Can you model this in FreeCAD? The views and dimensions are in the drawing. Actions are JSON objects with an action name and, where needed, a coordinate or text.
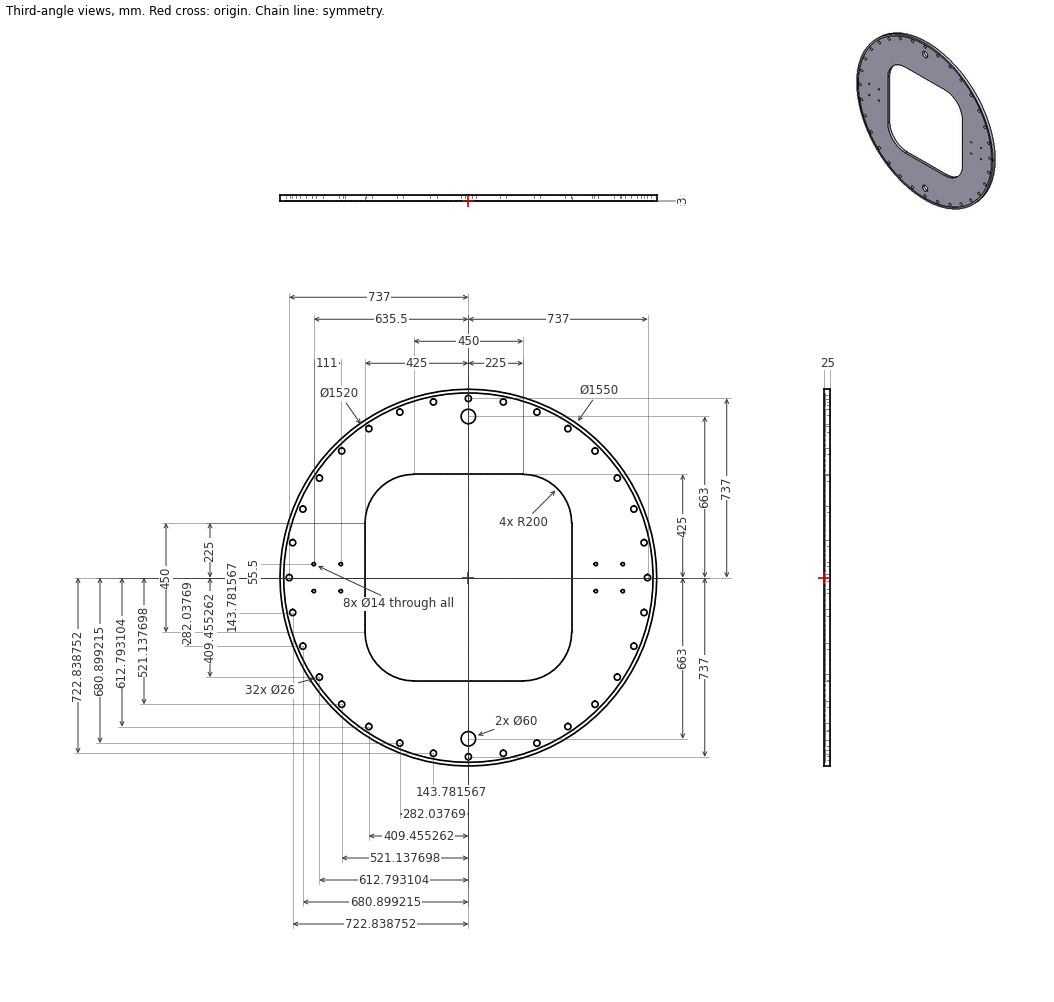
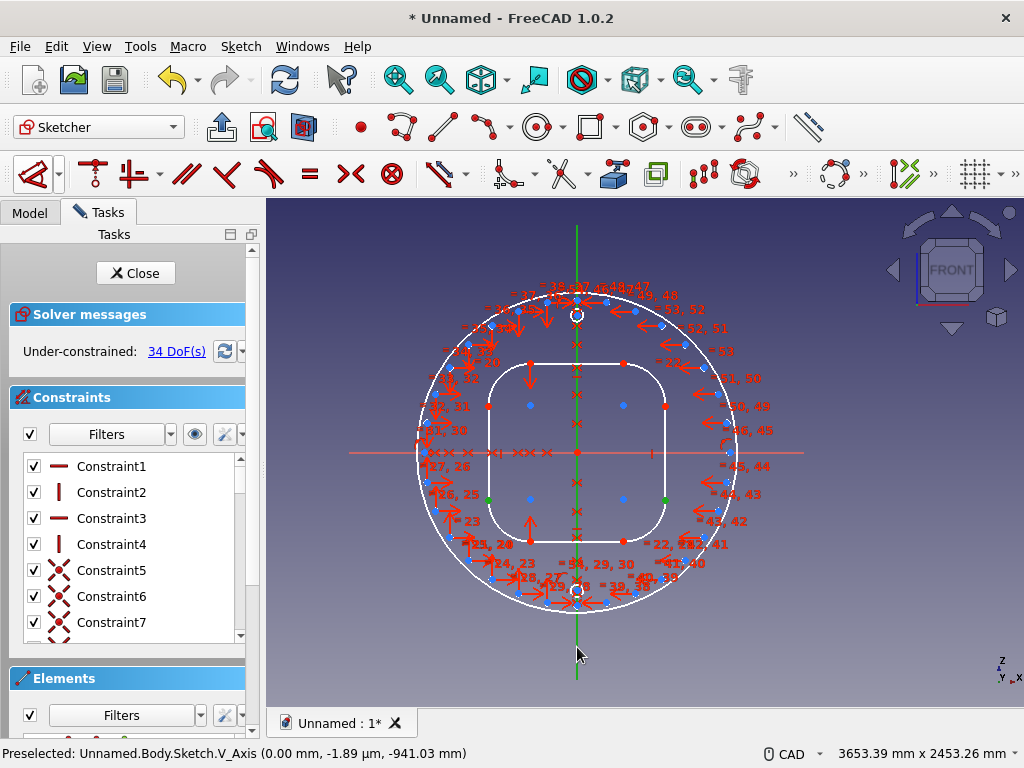
{"action": "left_click", "coordinate": [351, 174]}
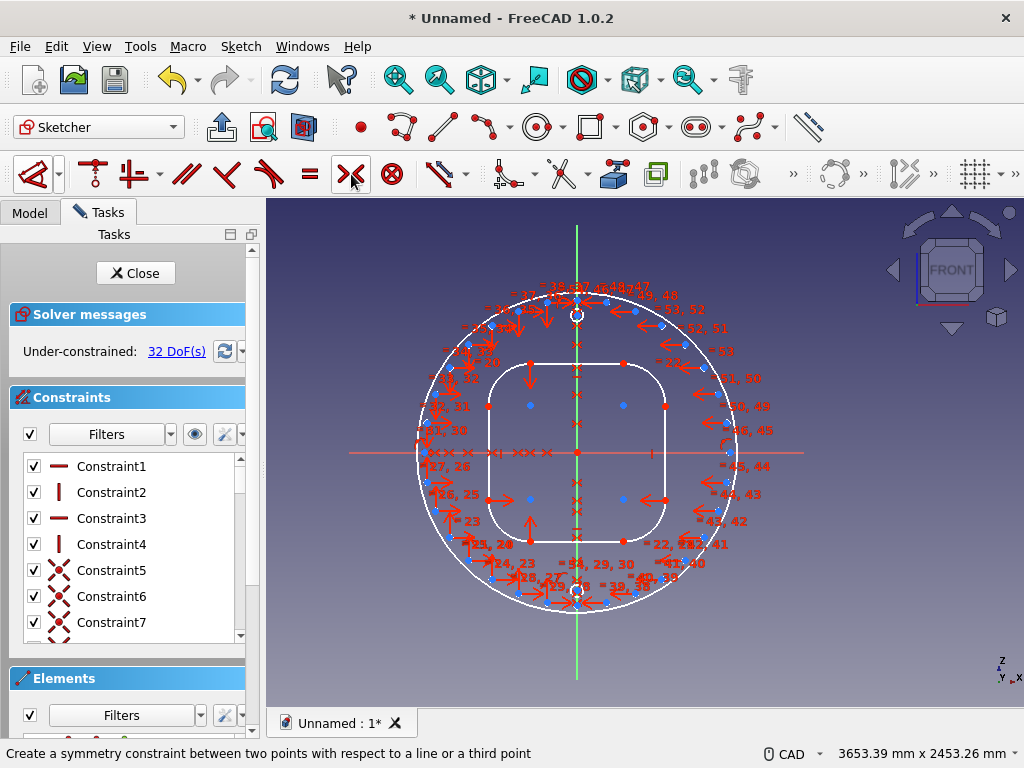
{"action": "left_click", "coordinate": [32, 174]}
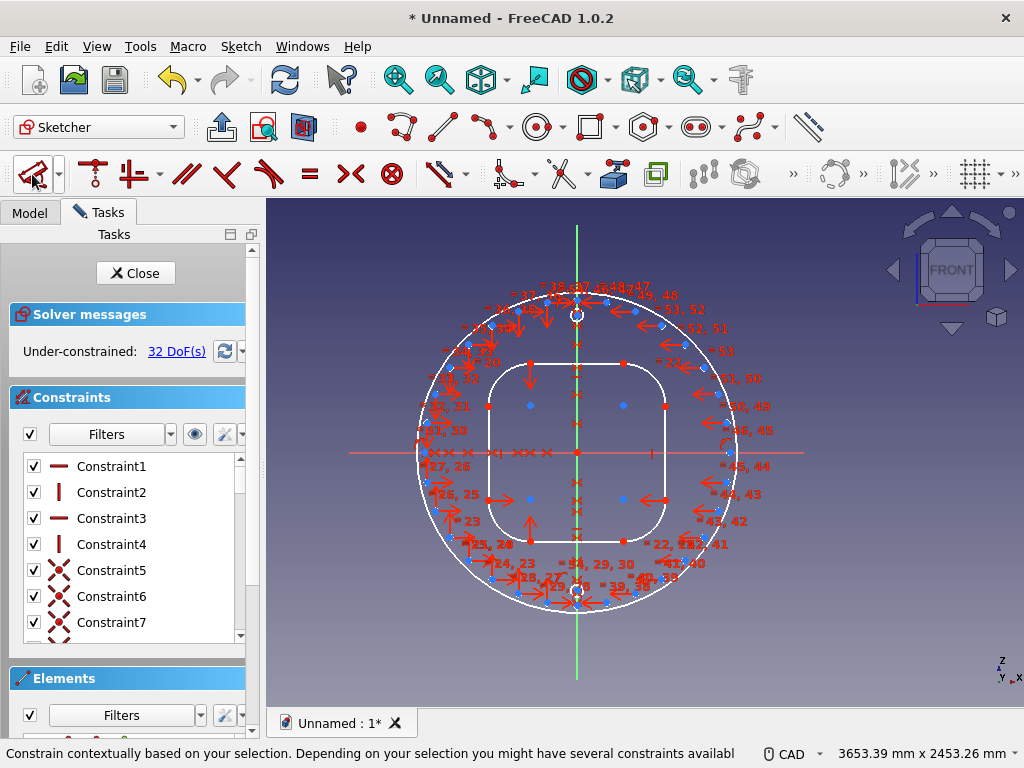
{"action": "left_click", "coordinate": [511, 369]}
{"action": "left_click", "coordinate": [531, 332]}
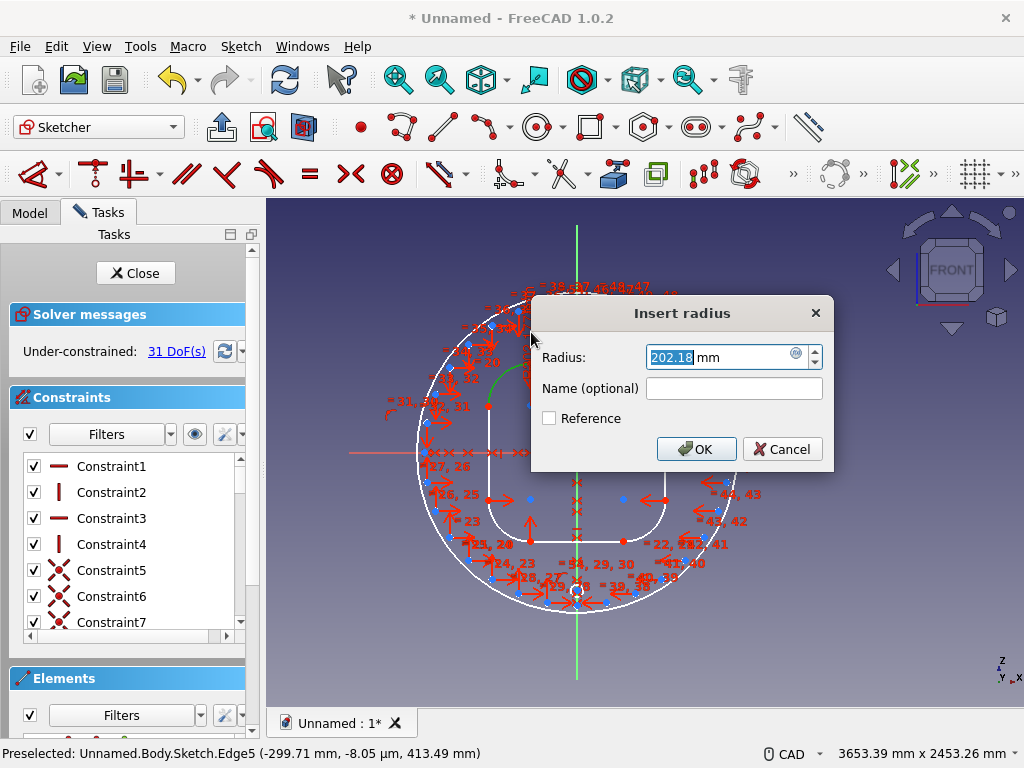
{"action": "type", "text": "200"}
{"action": "key", "text": "Return"}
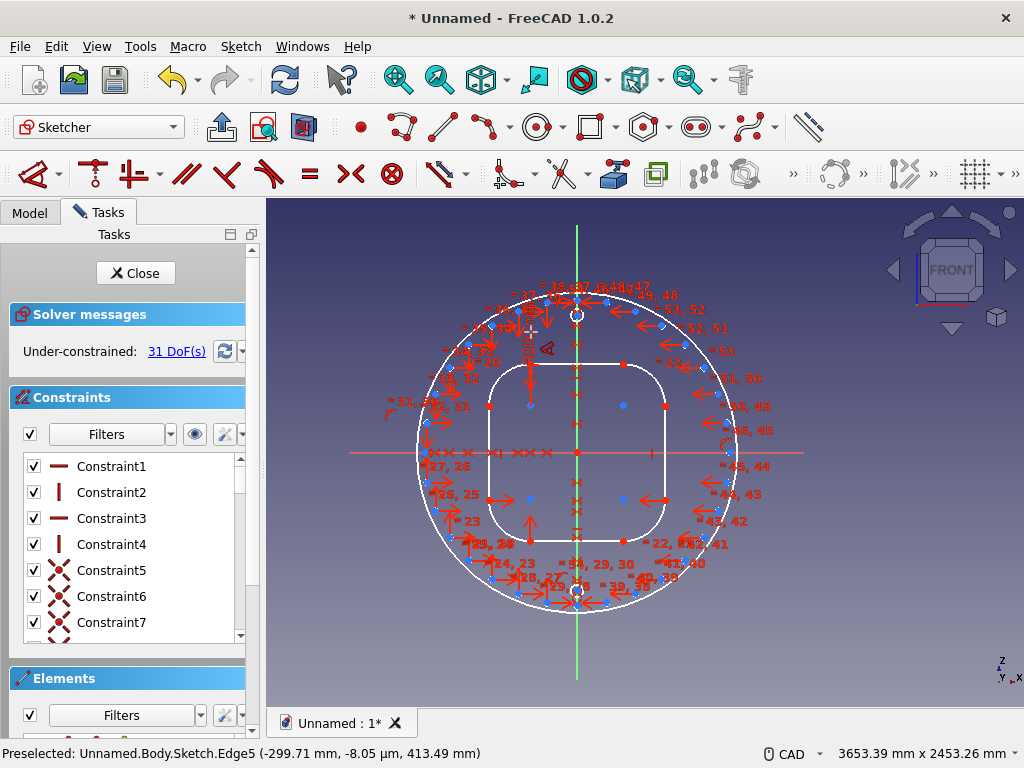
{"action": "scroll", "coordinate": [690, 339], "scroll_direction": "up", "scroll_amount": 6}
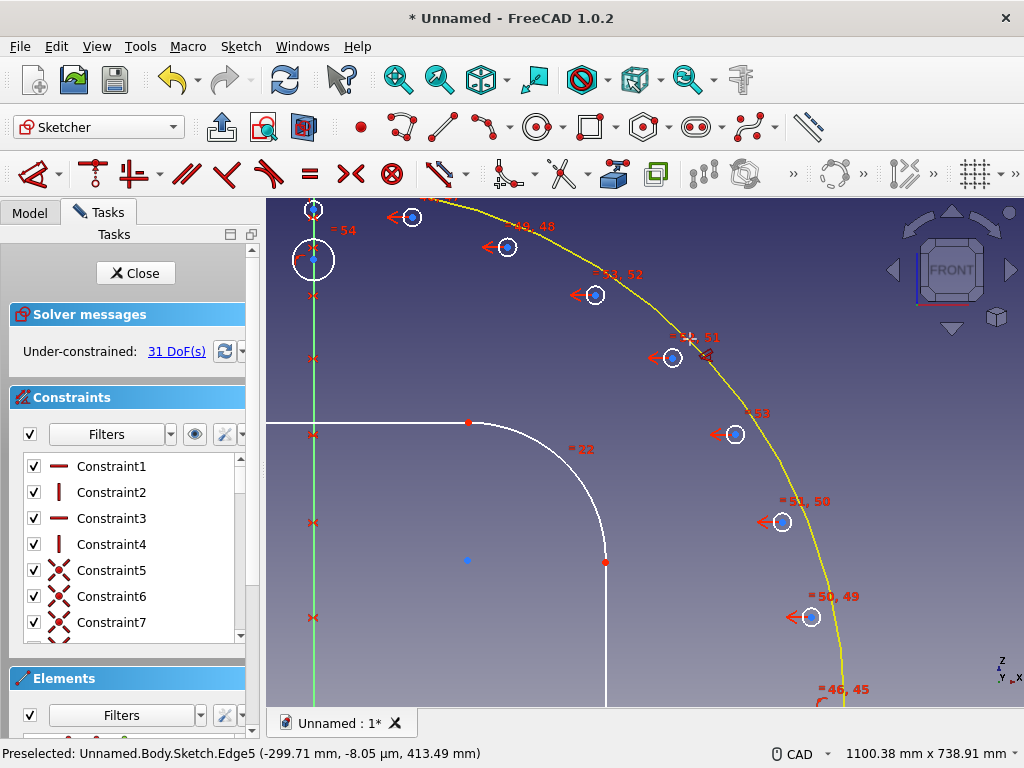
{"action": "left_click", "coordinate": [688, 339]}
{"action": "left_click", "coordinate": [711, 316]}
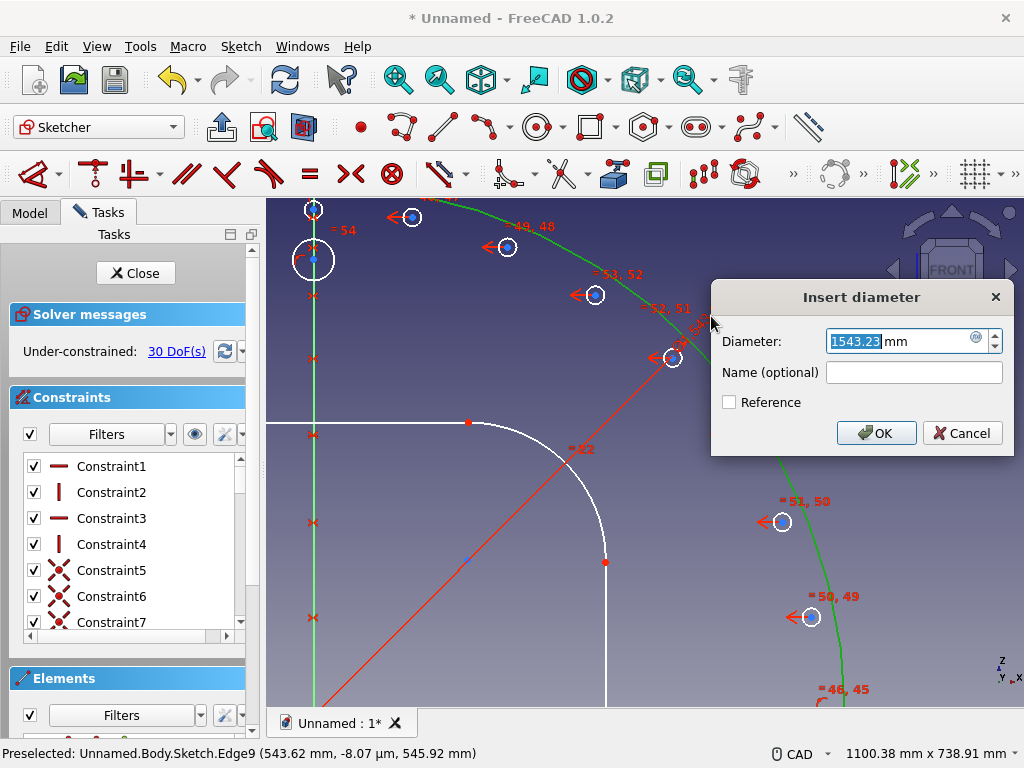
{"action": "type", "text": "1550"}
{"action": "key", "text": "Return"}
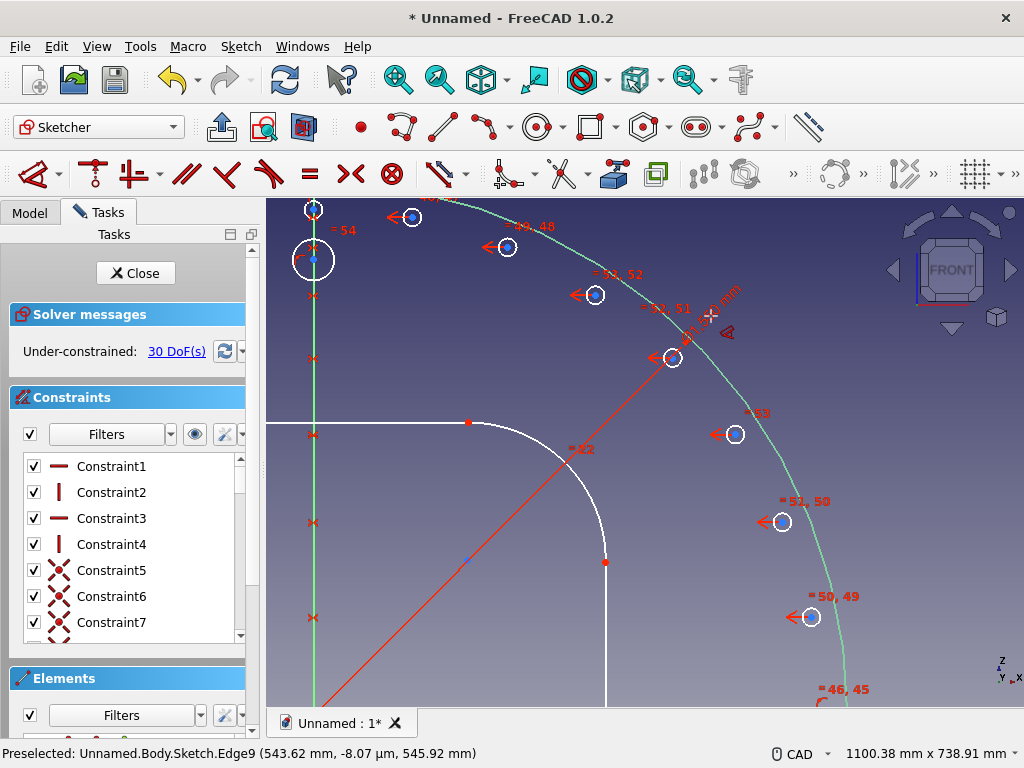
{"action": "scroll", "coordinate": [690, 339], "scroll_direction": "down", "scroll_amount": 6}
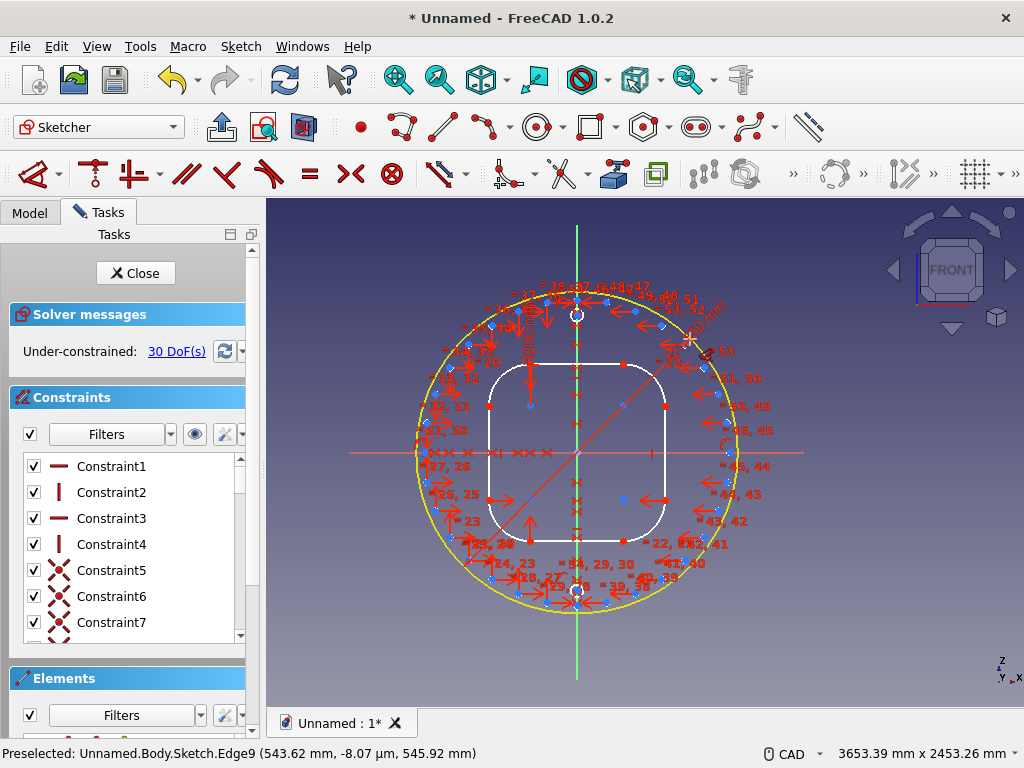
{"action": "scroll", "coordinate": [450, 535], "scroll_direction": "up", "scroll_amount": 10}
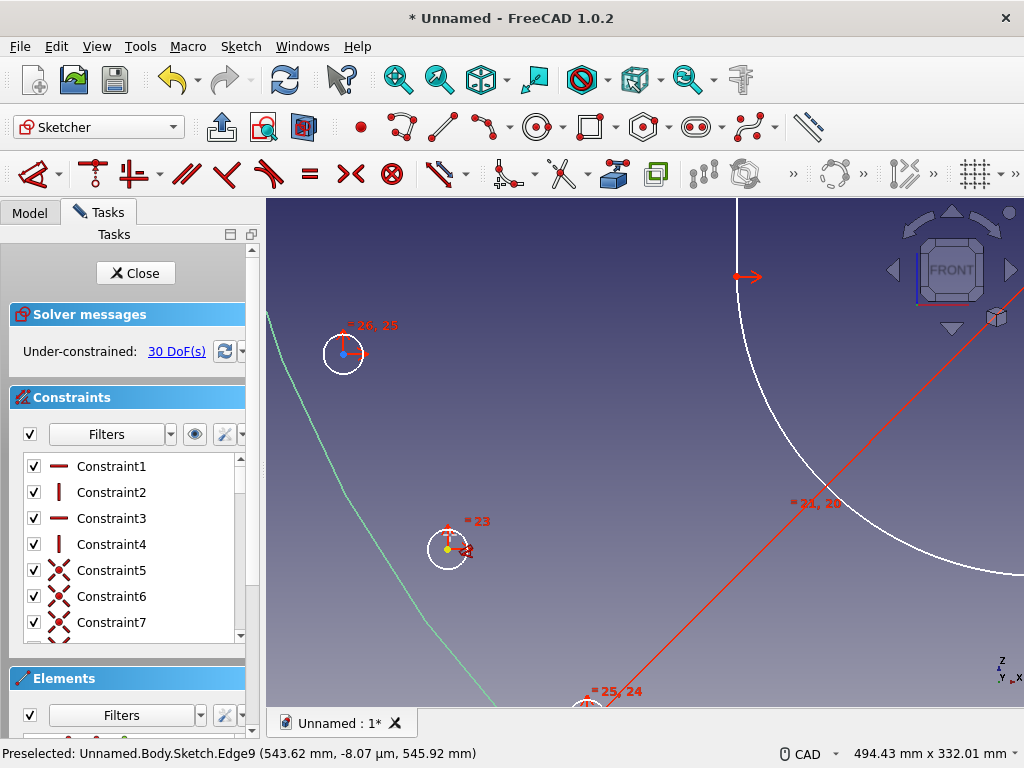
{"action": "left_click", "coordinate": [448, 530]}
{"action": "left_click", "coordinate": [448, 498]}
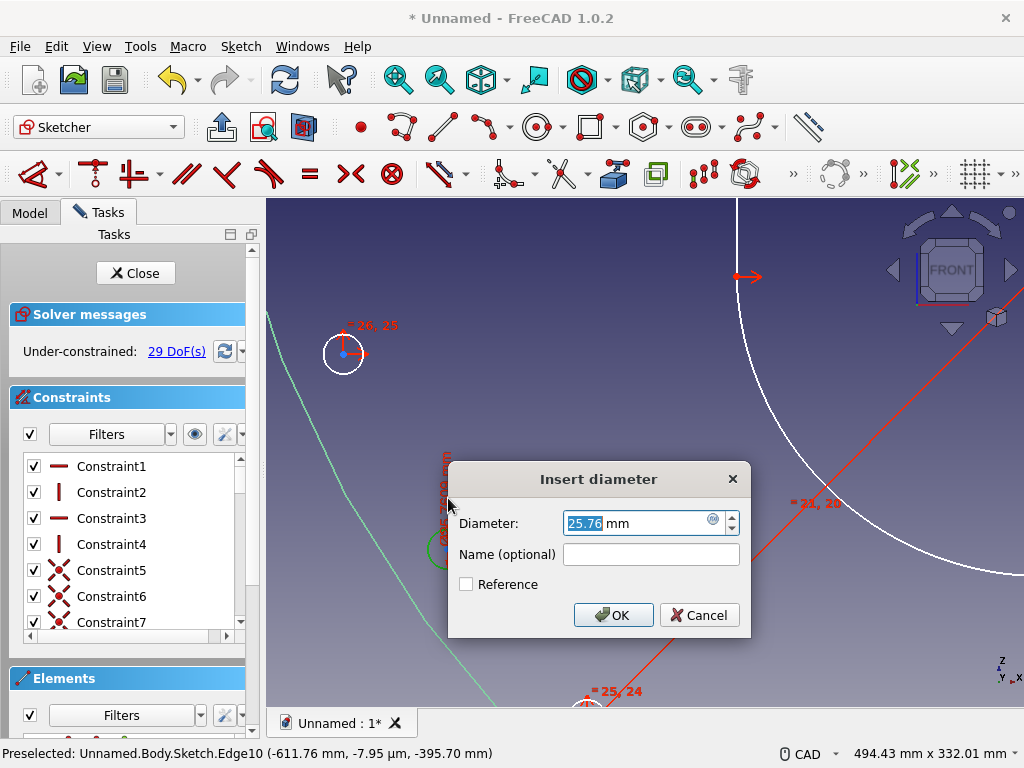
{"action": "type", "text": "26"}
{"action": "key", "text": "Return"}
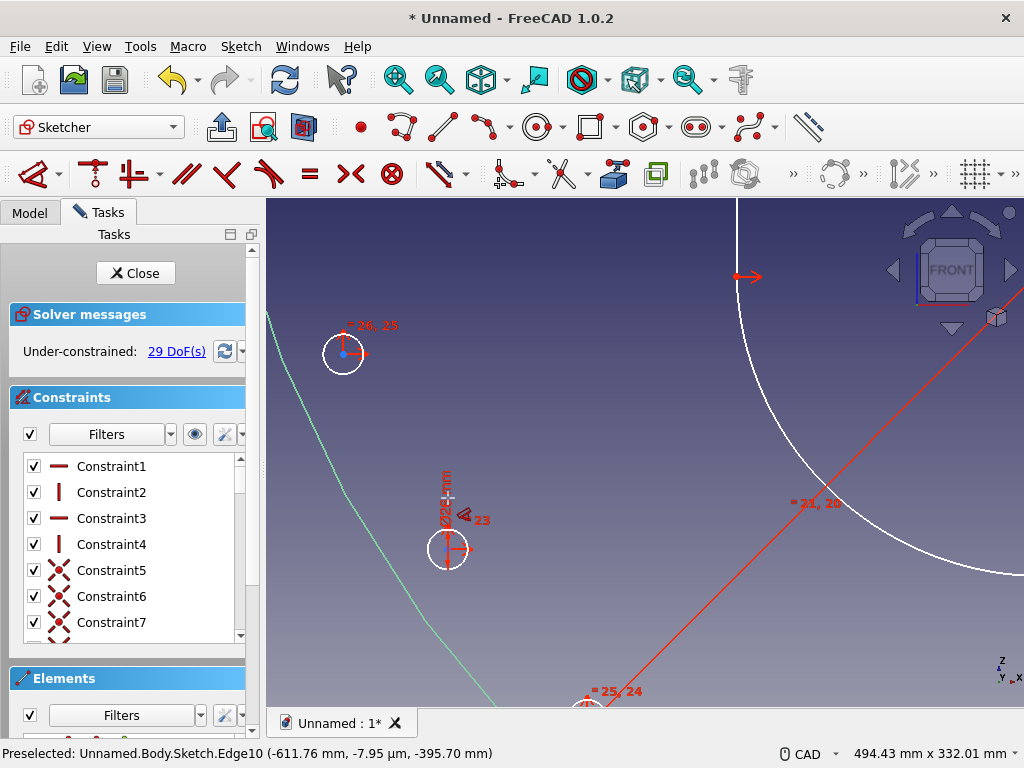
{"action": "scroll", "coordinate": [450, 535], "scroll_direction": "down", "scroll_amount": 10}